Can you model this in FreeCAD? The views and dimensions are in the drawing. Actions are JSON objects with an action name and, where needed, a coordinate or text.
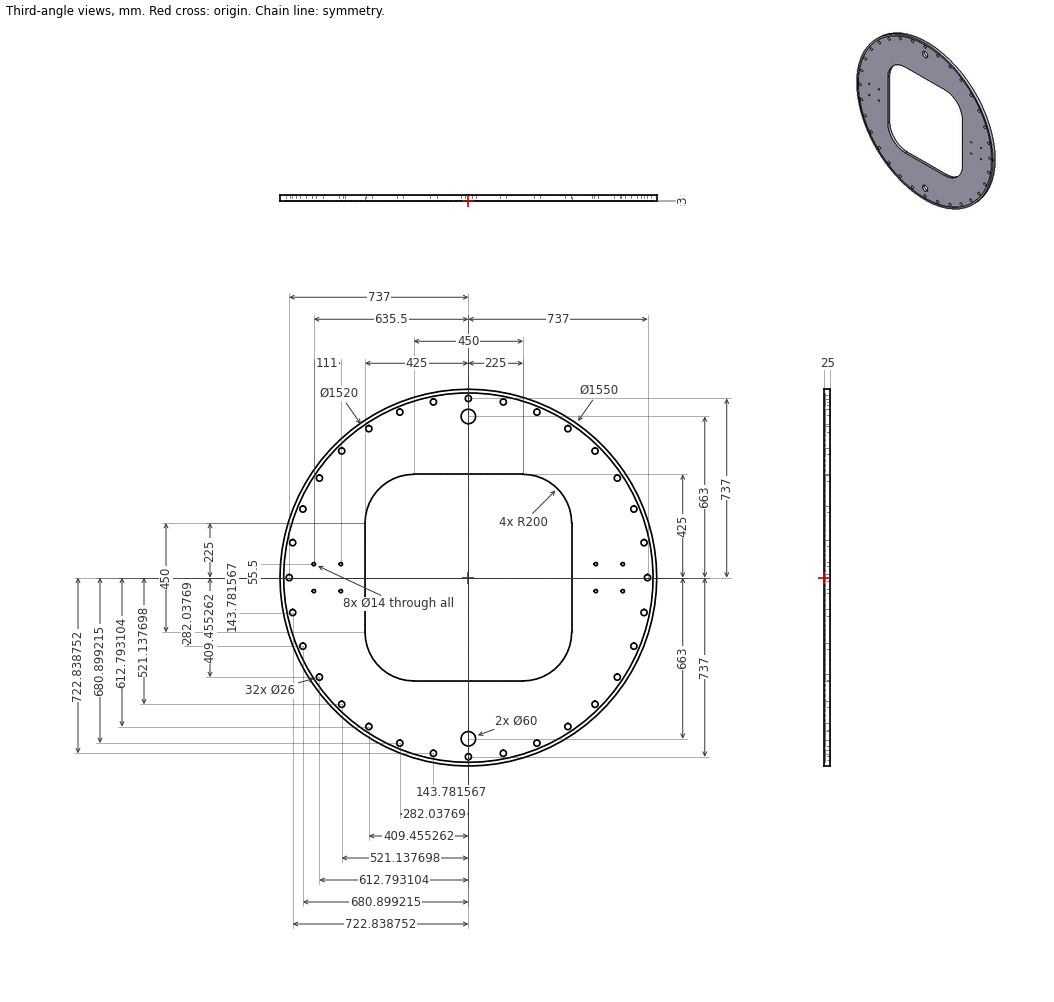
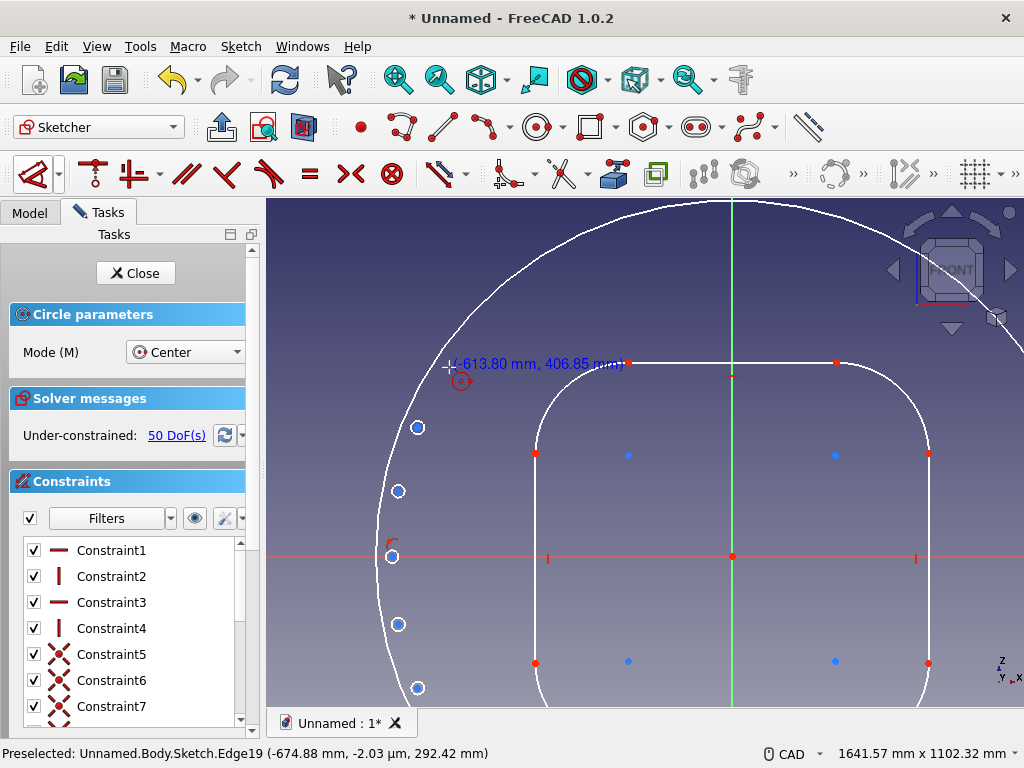
{"action": "left_click", "coordinate": [449, 368]}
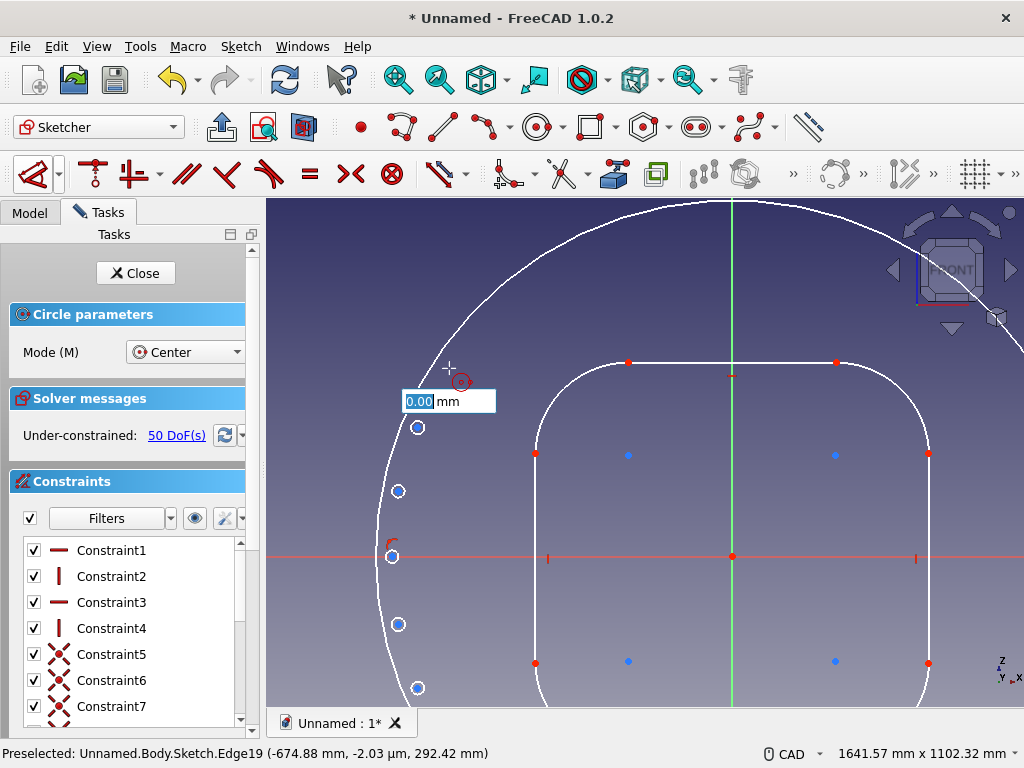
{"action": "scroll", "coordinate": [453, 363], "scroll_direction": "up", "scroll_amount": 5}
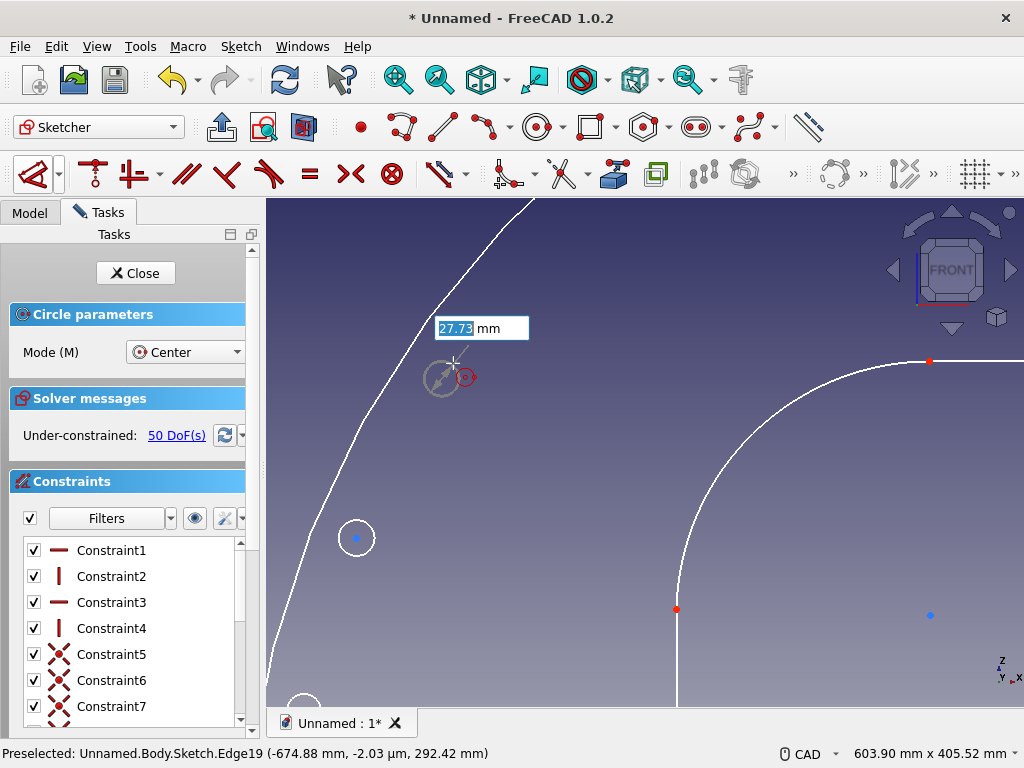
{"action": "left_click", "coordinate": [454, 363]}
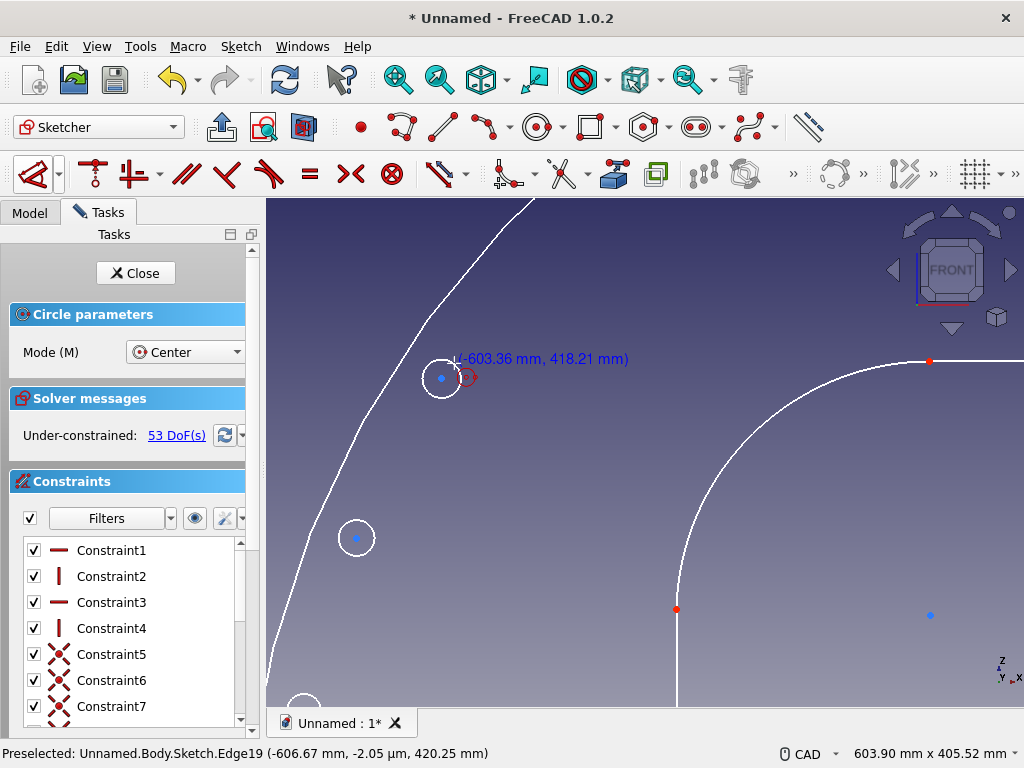
{"action": "scroll", "coordinate": [557, 235], "scroll_direction": "up", "scroll_amount": 2}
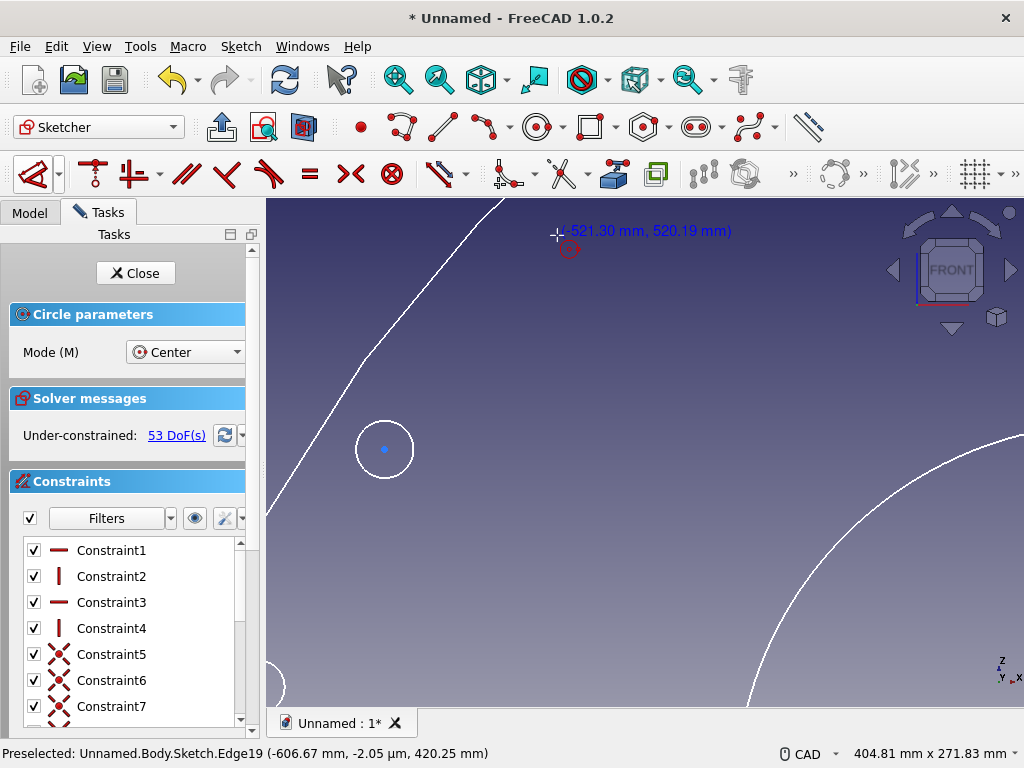
{"action": "scroll", "coordinate": [457, 358], "scroll_direction": "down", "scroll_amount": 11}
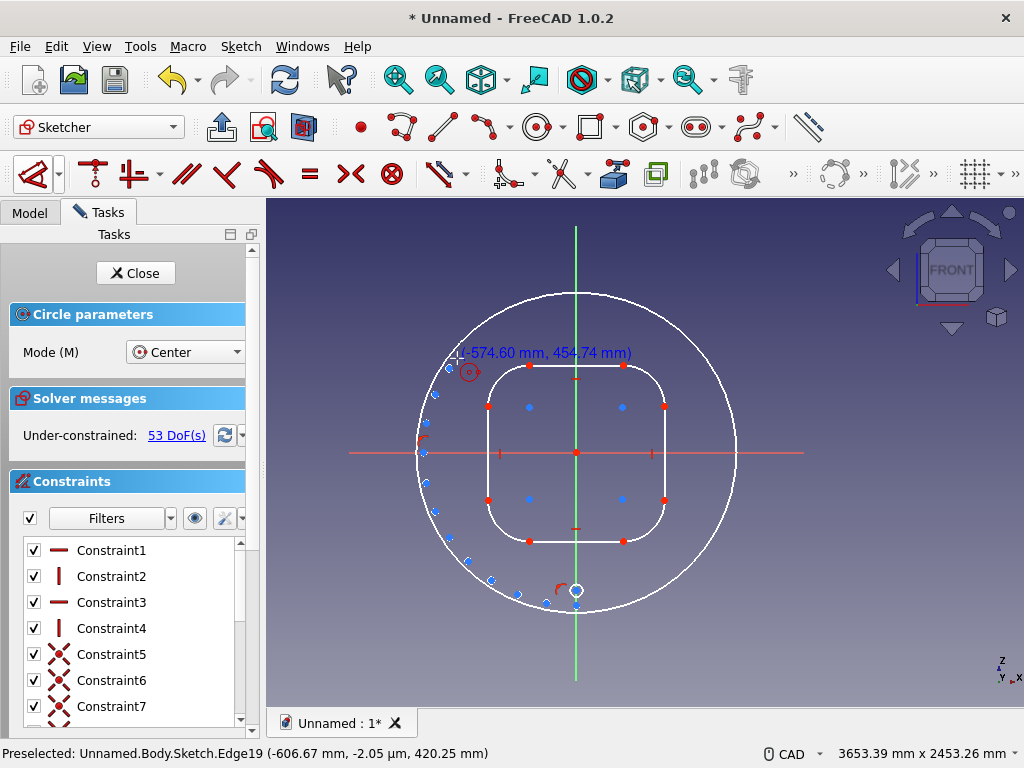
{"action": "scroll", "coordinate": [468, 345], "scroll_direction": "up", "scroll_amount": 4}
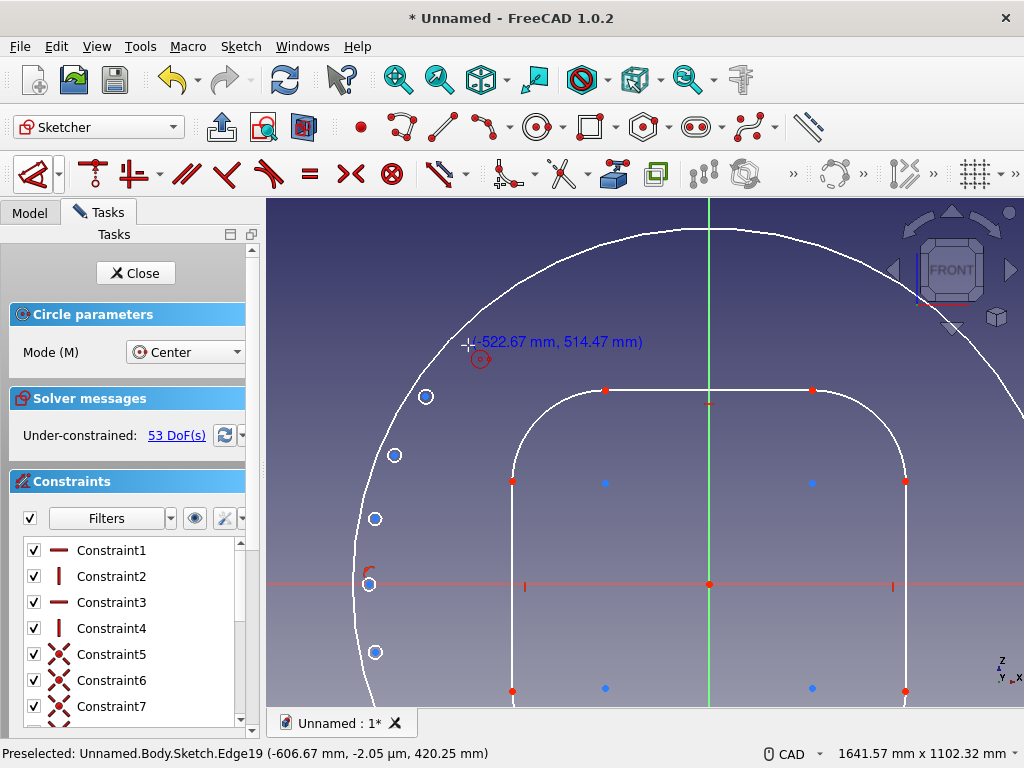
{"action": "left_click", "coordinate": [468, 344]}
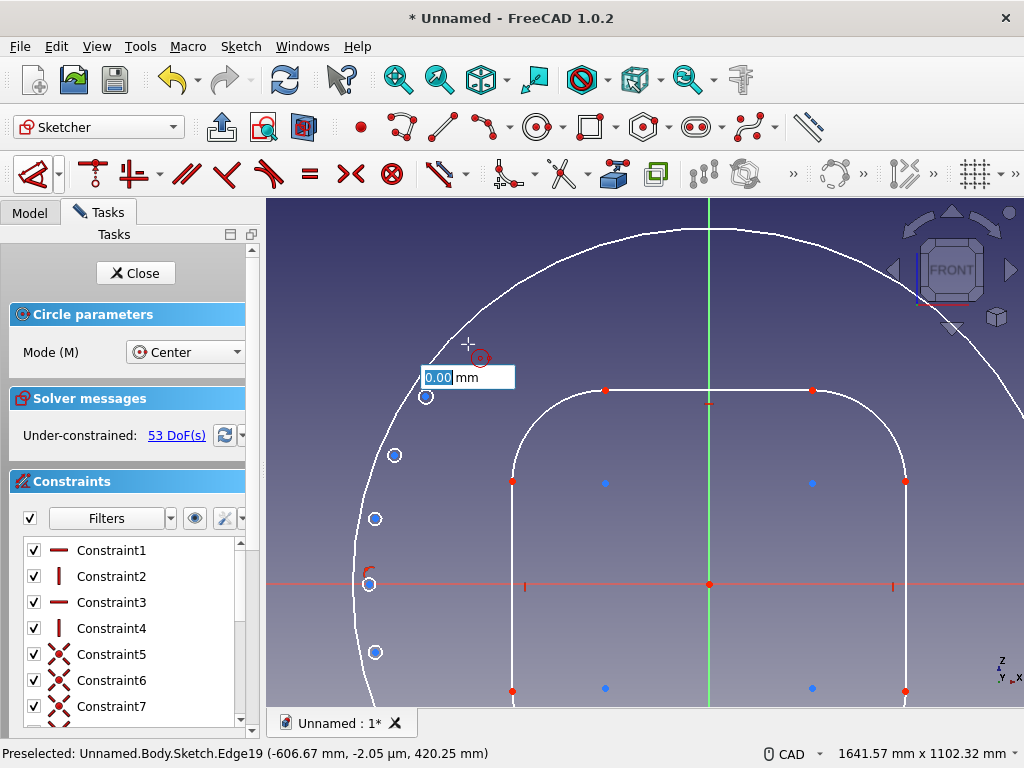
{"action": "scroll", "coordinate": [473, 340], "scroll_direction": "up", "scroll_amount": 5}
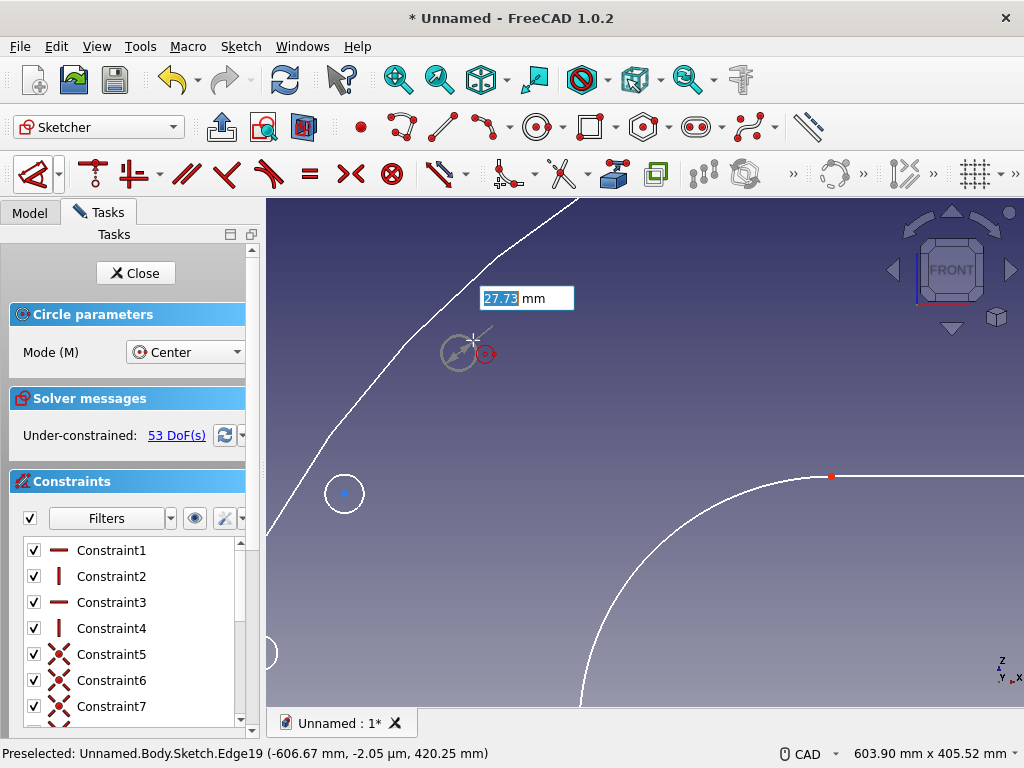
{"action": "left_click", "coordinate": [472, 338]}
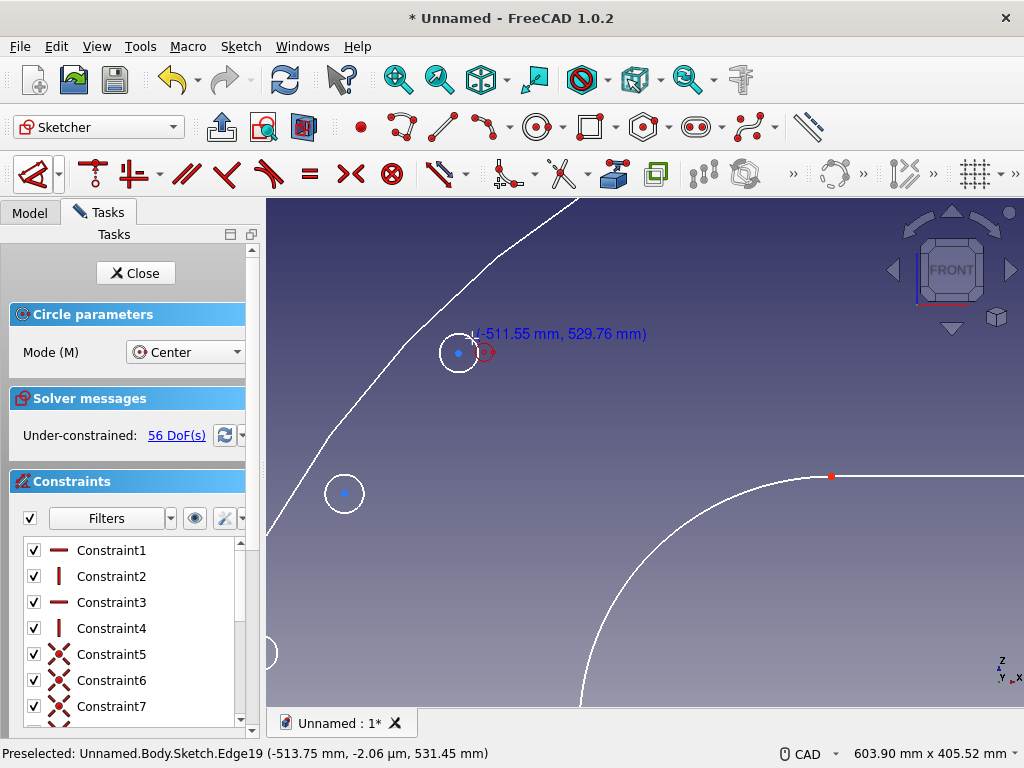
{"action": "scroll", "coordinate": [600, 235], "scroll_direction": "up", "scroll_amount": 2}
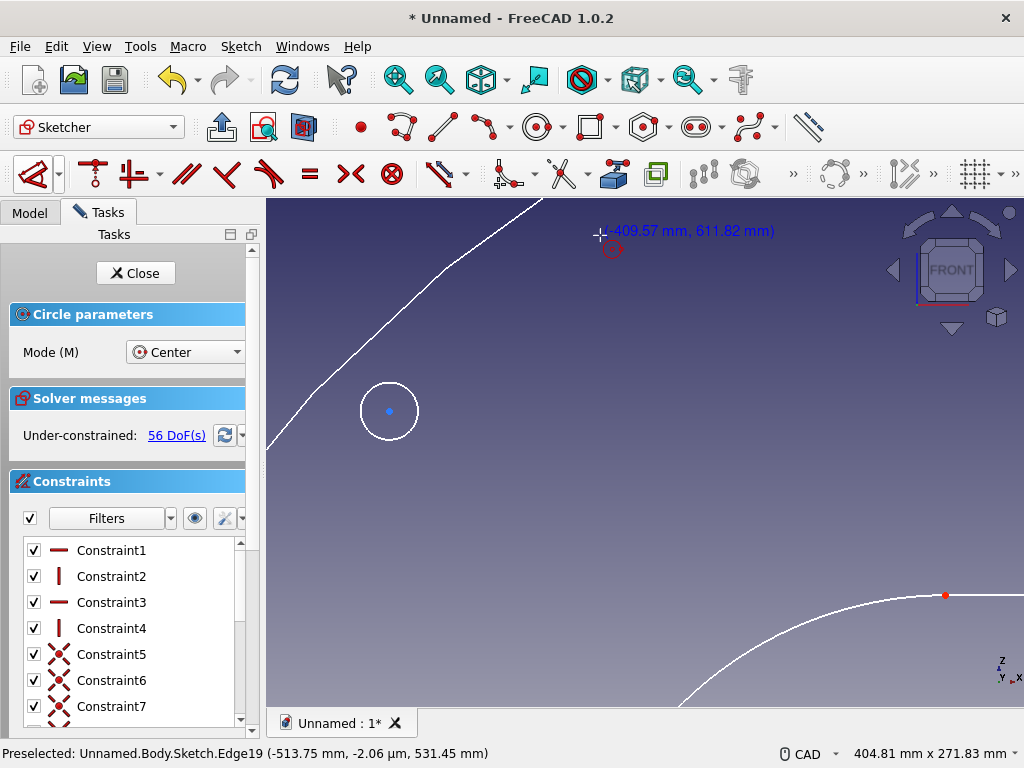
{"action": "scroll", "coordinate": [478, 337], "scroll_direction": "down", "scroll_amount": 11}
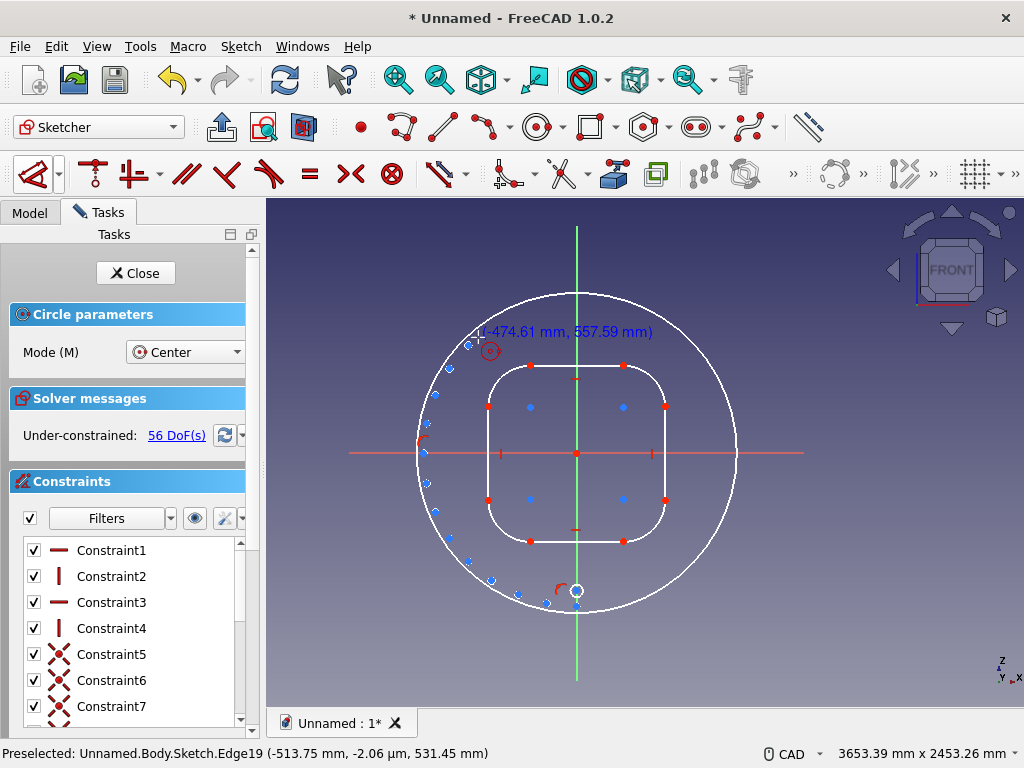
{"action": "scroll", "coordinate": [492, 326], "scroll_direction": "up", "scroll_amount": 4}